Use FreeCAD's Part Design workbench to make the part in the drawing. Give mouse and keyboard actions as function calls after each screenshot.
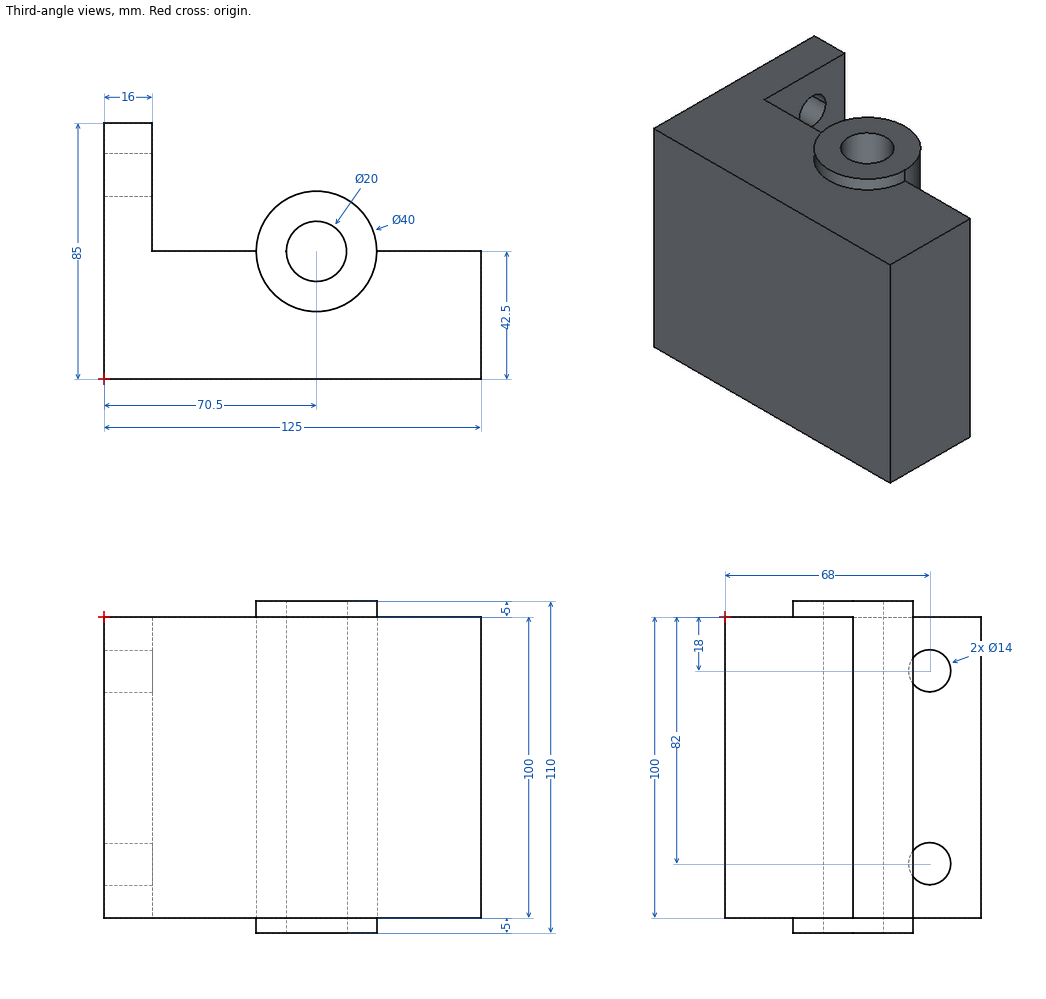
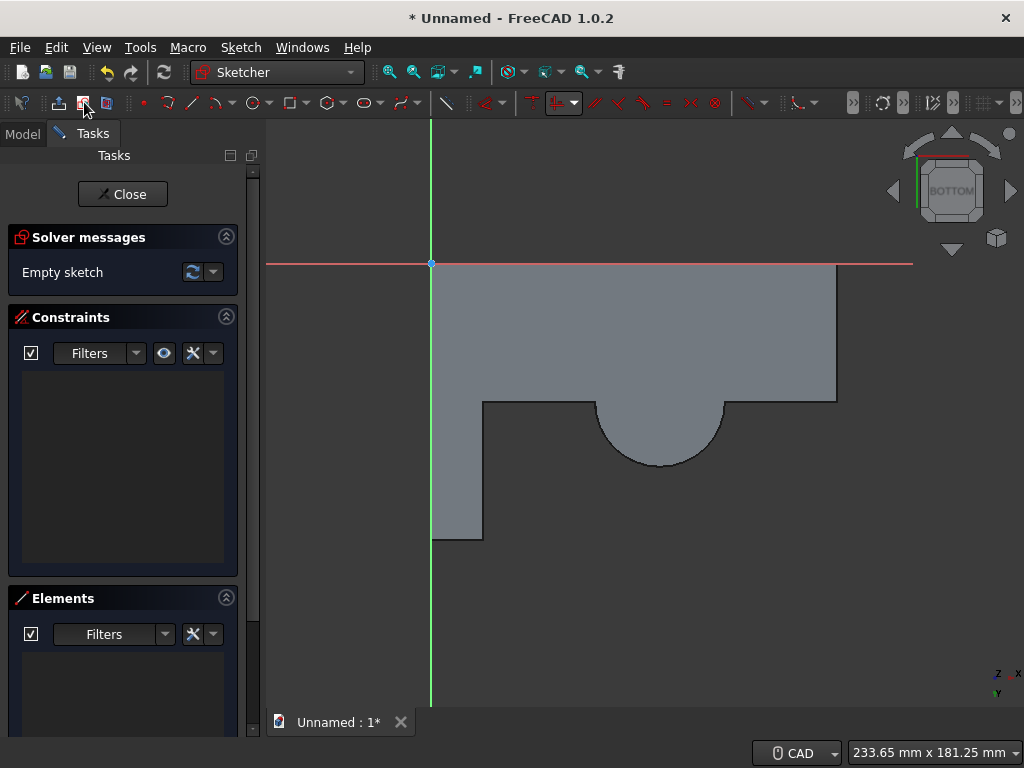
scroll(581, 269, up, 2)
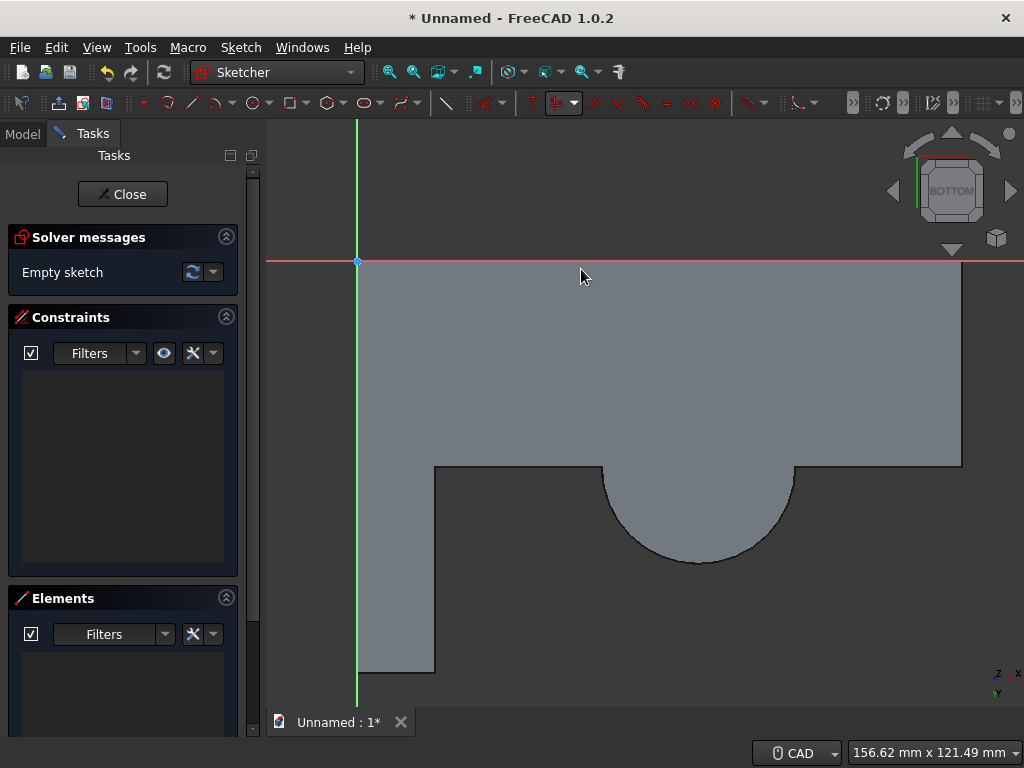
key(g)
key(c)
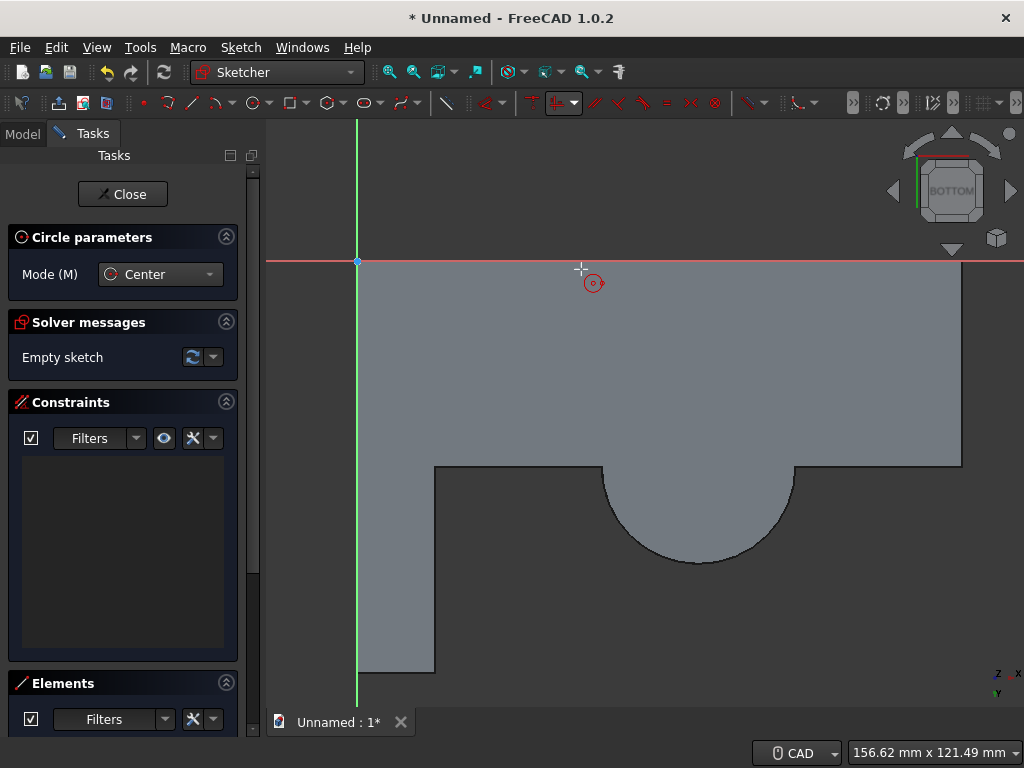
click(699, 467)
move(767, 399)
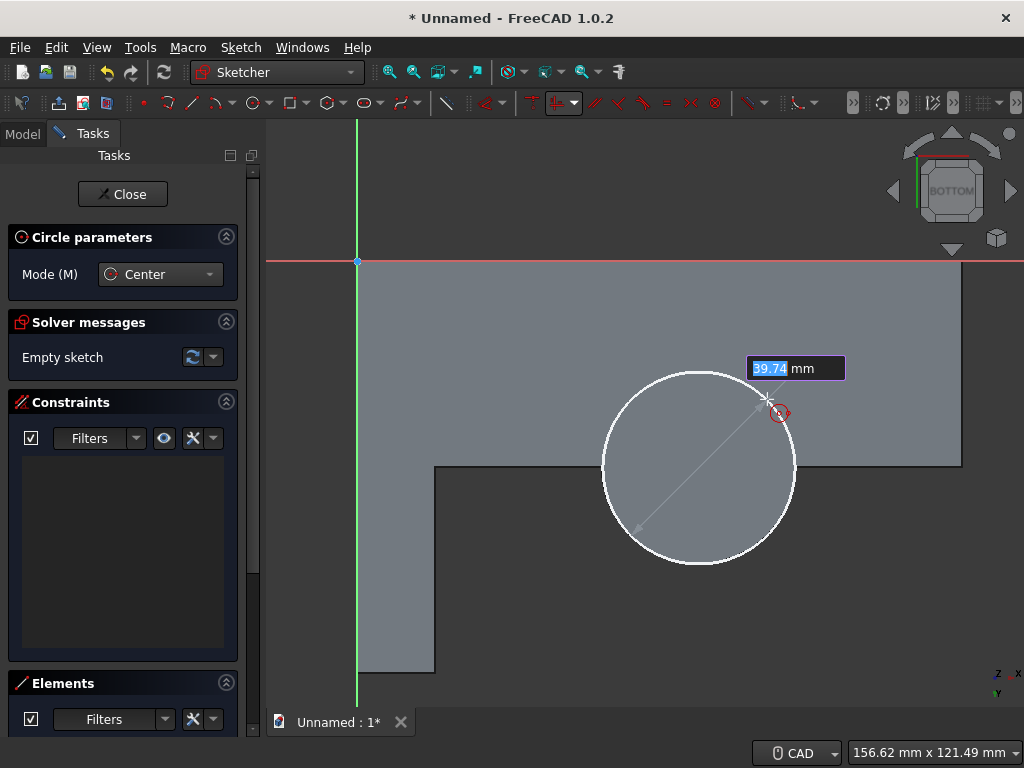
text(40)
key(Return)
key(Escape)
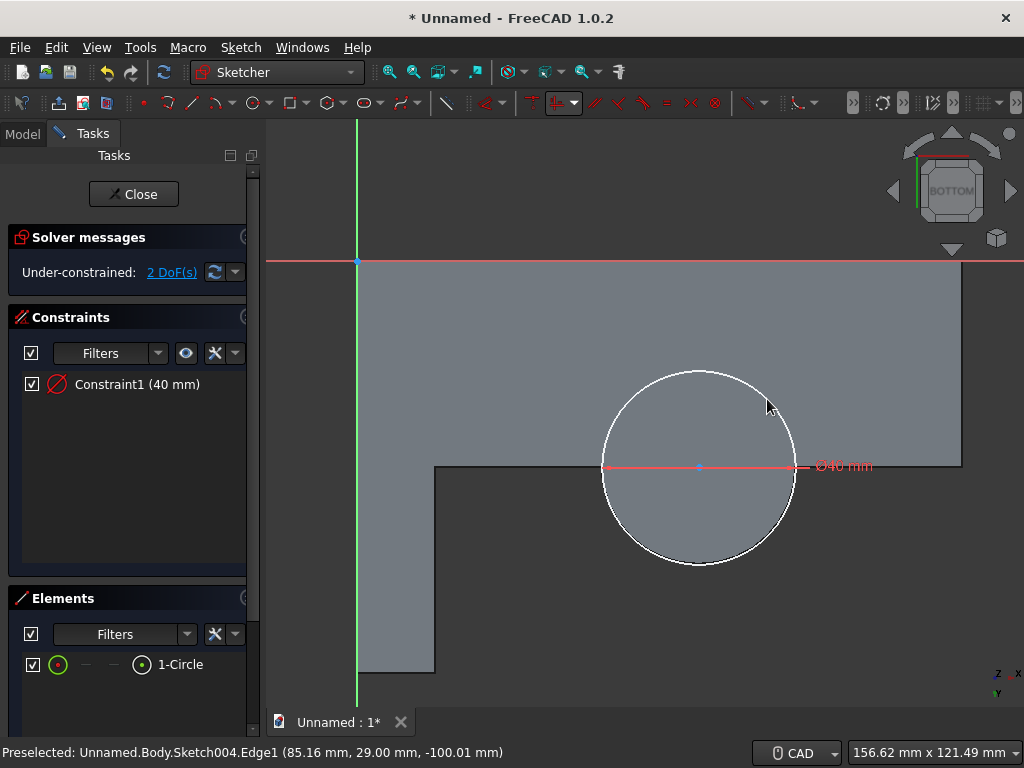
click(486, 104)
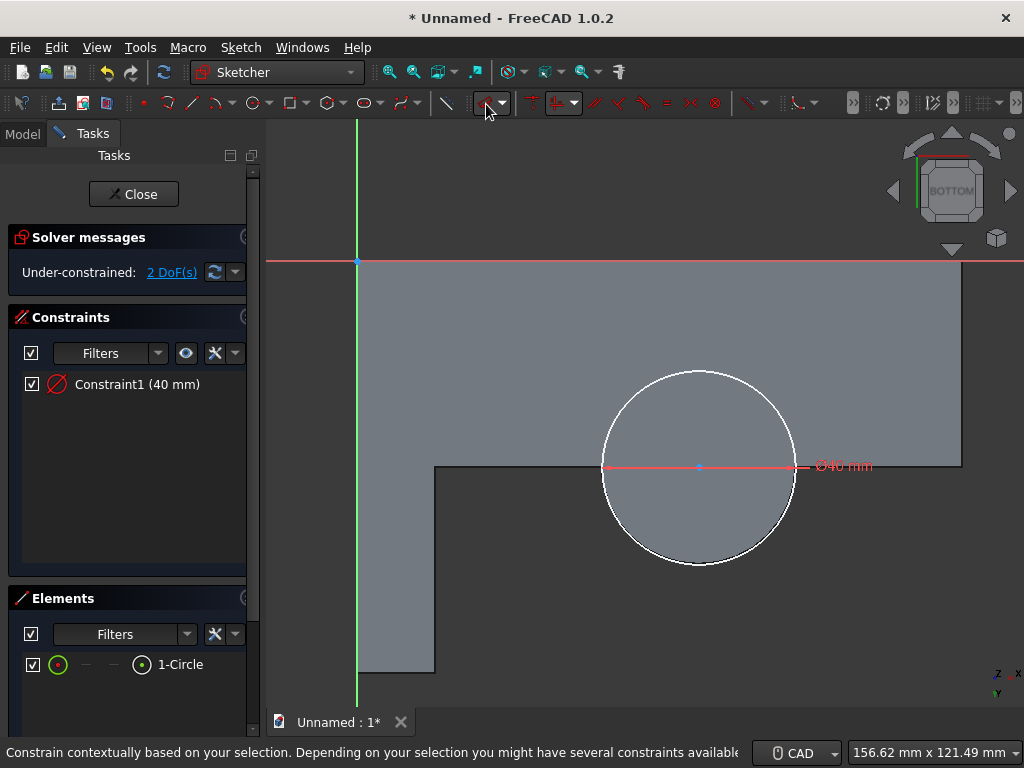
click(699, 468)
click(528, 227)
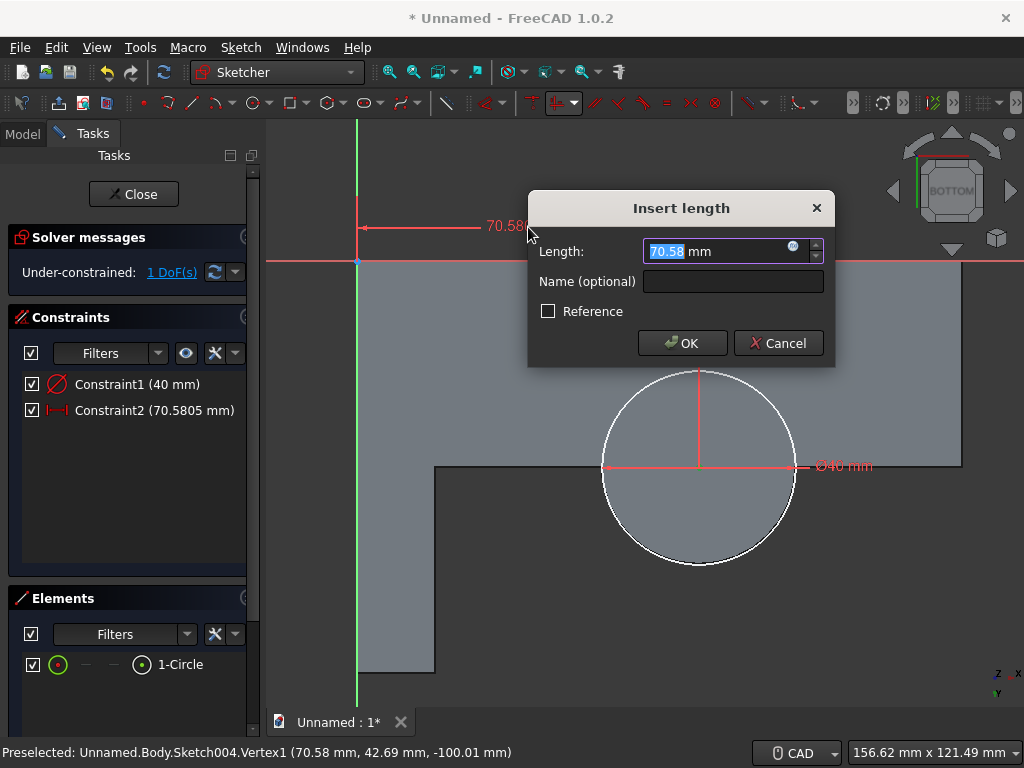
text(70.5)
key(Return)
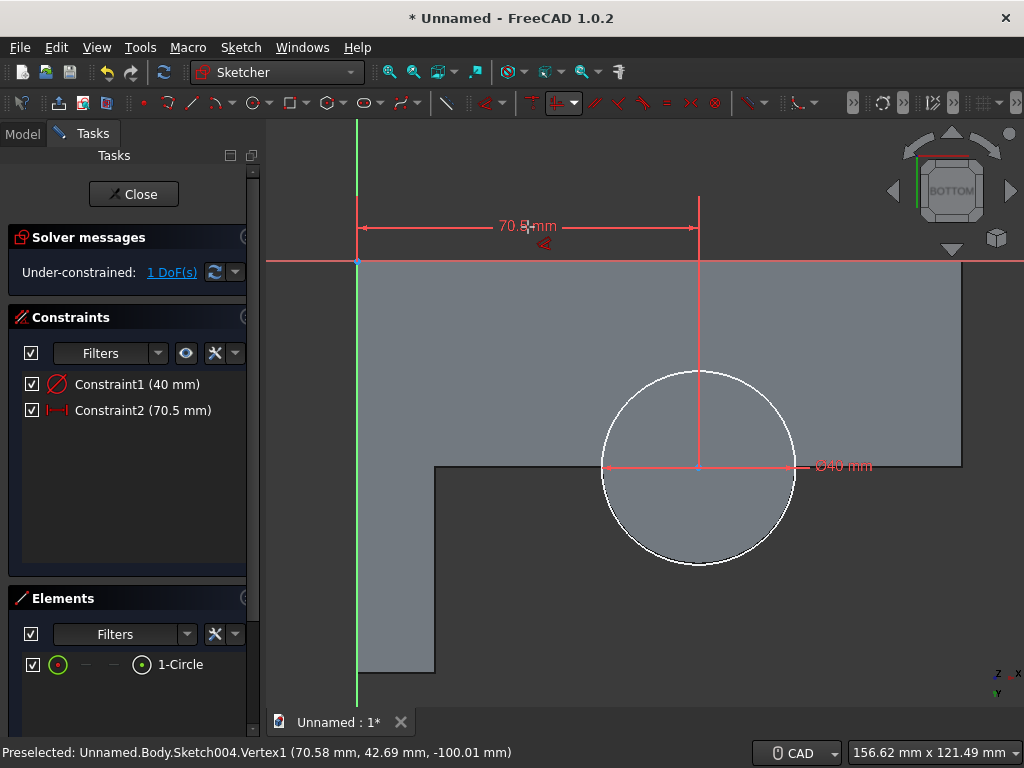
click(699, 468)
click(323, 365)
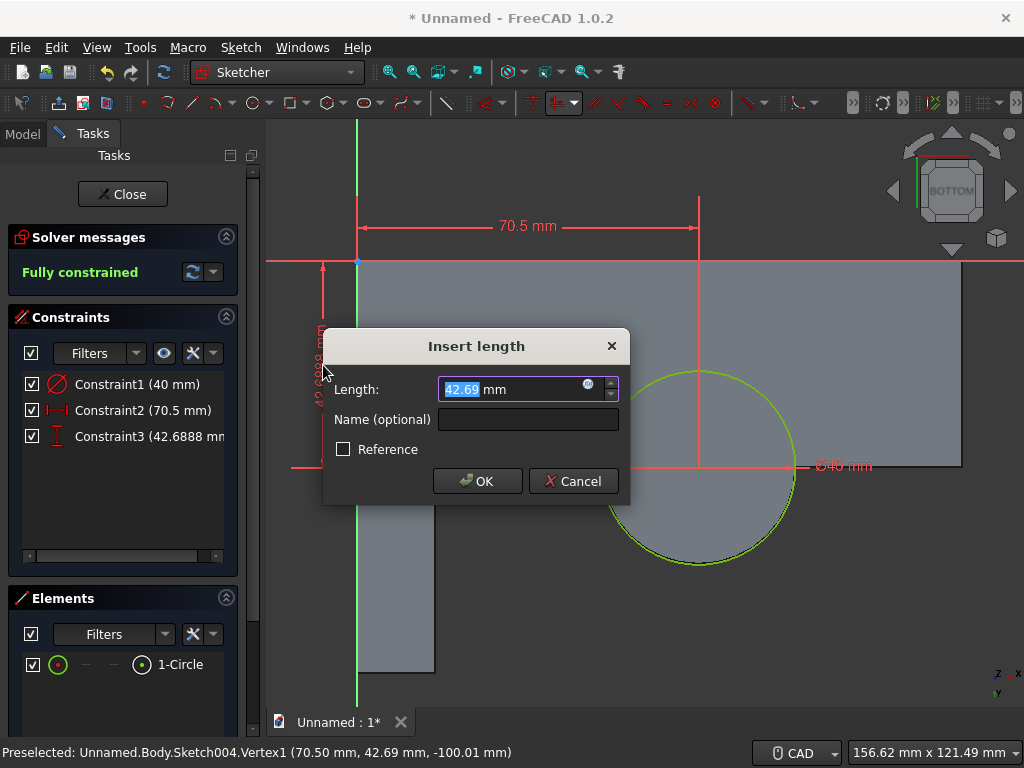
text(42.5)
key(Return)
key(Escape)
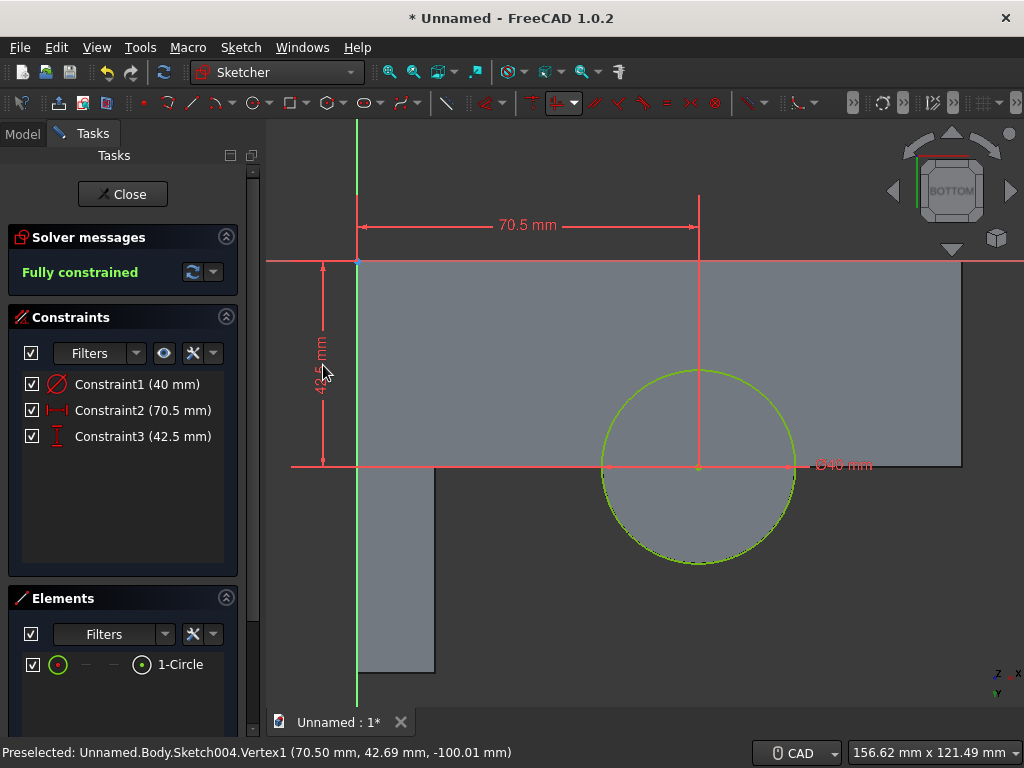
click(123, 194)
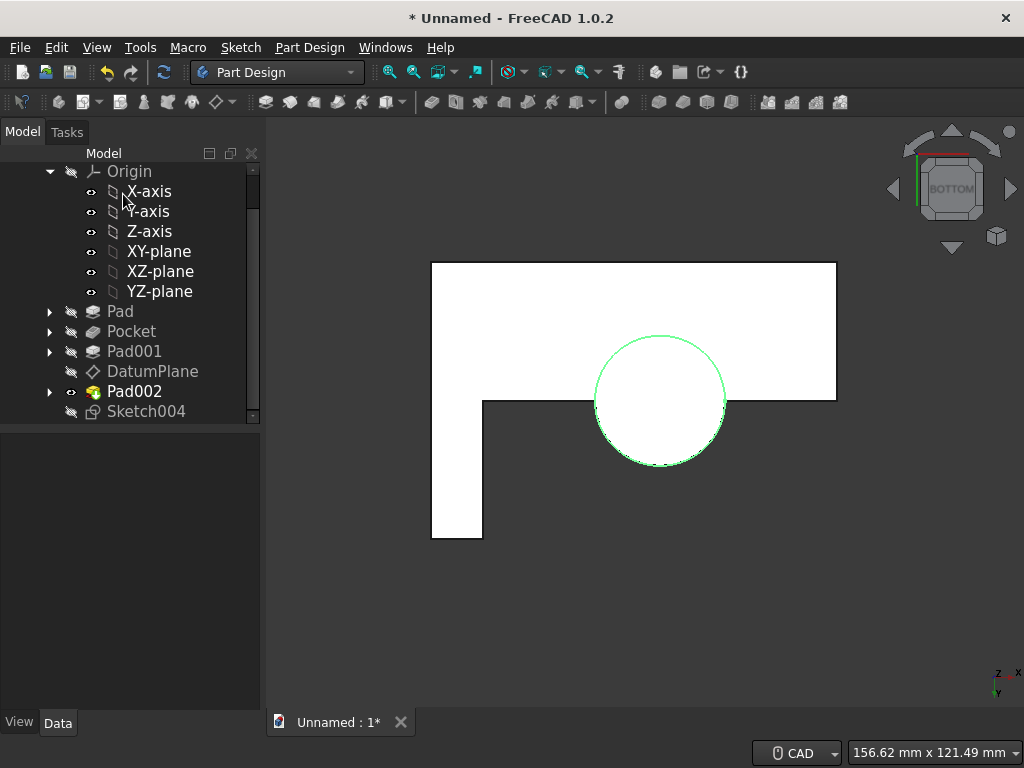
click(266, 102)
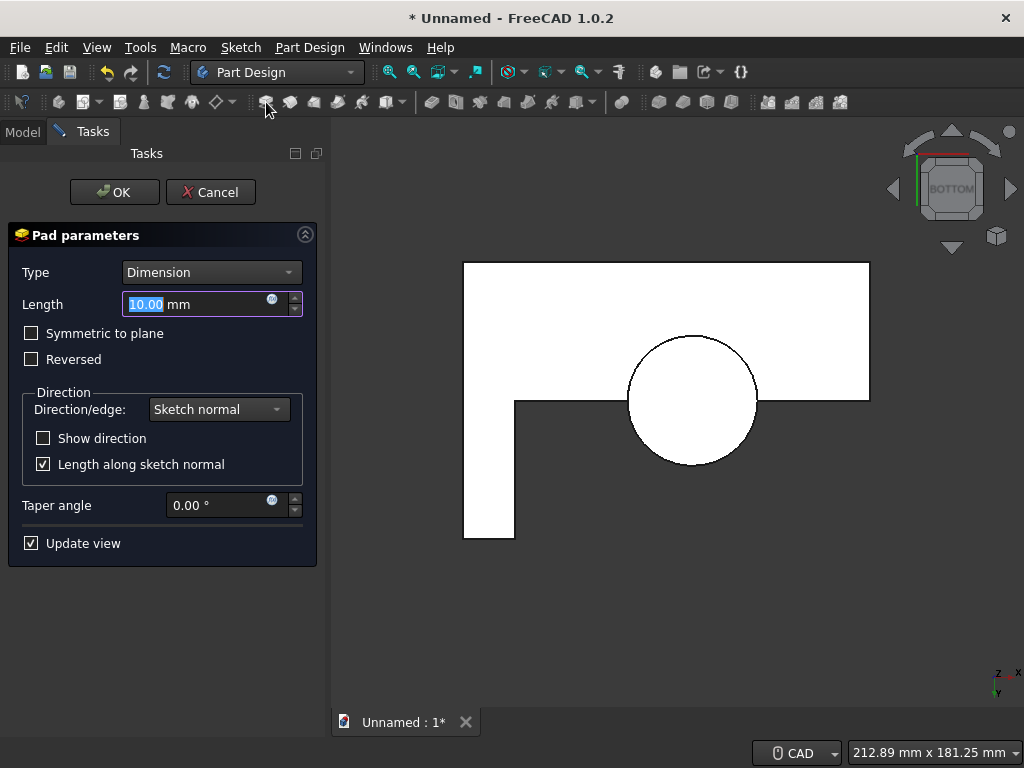
text(5)
key(Tab)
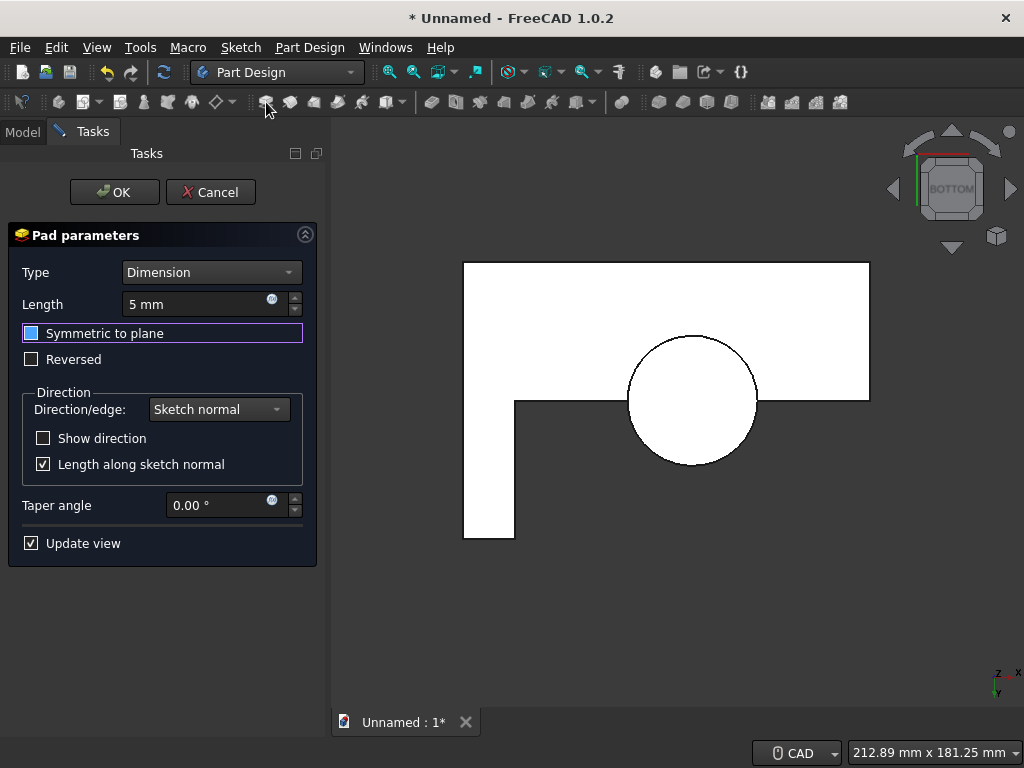
click(115, 192)